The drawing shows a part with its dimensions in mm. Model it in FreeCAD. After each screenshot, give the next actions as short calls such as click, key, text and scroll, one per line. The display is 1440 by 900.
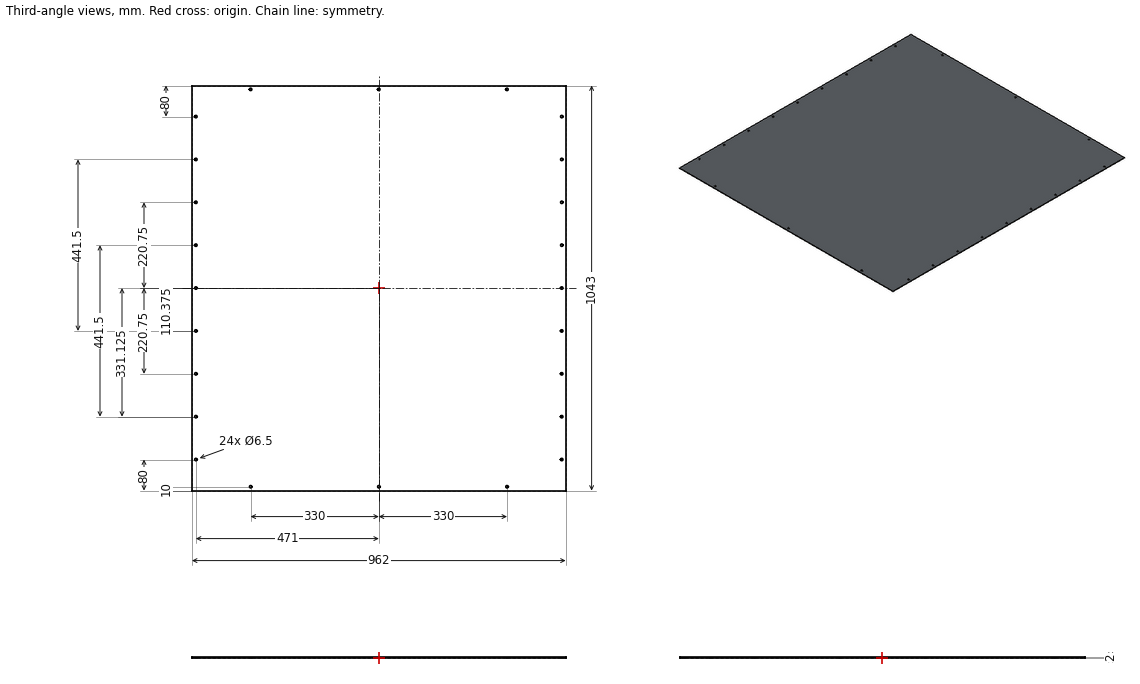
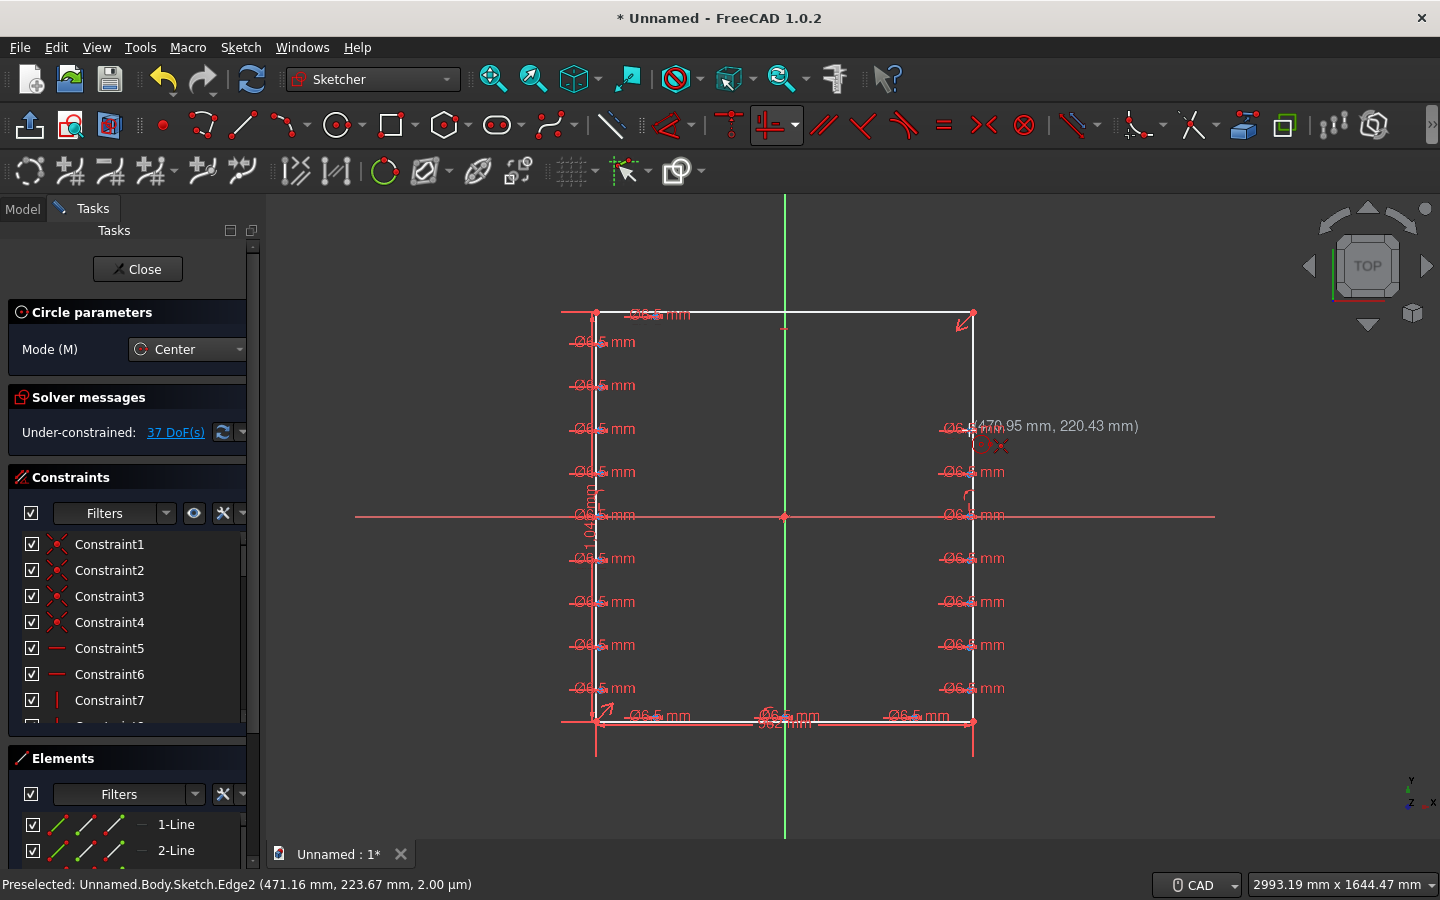
scroll(785, 316, up, 15)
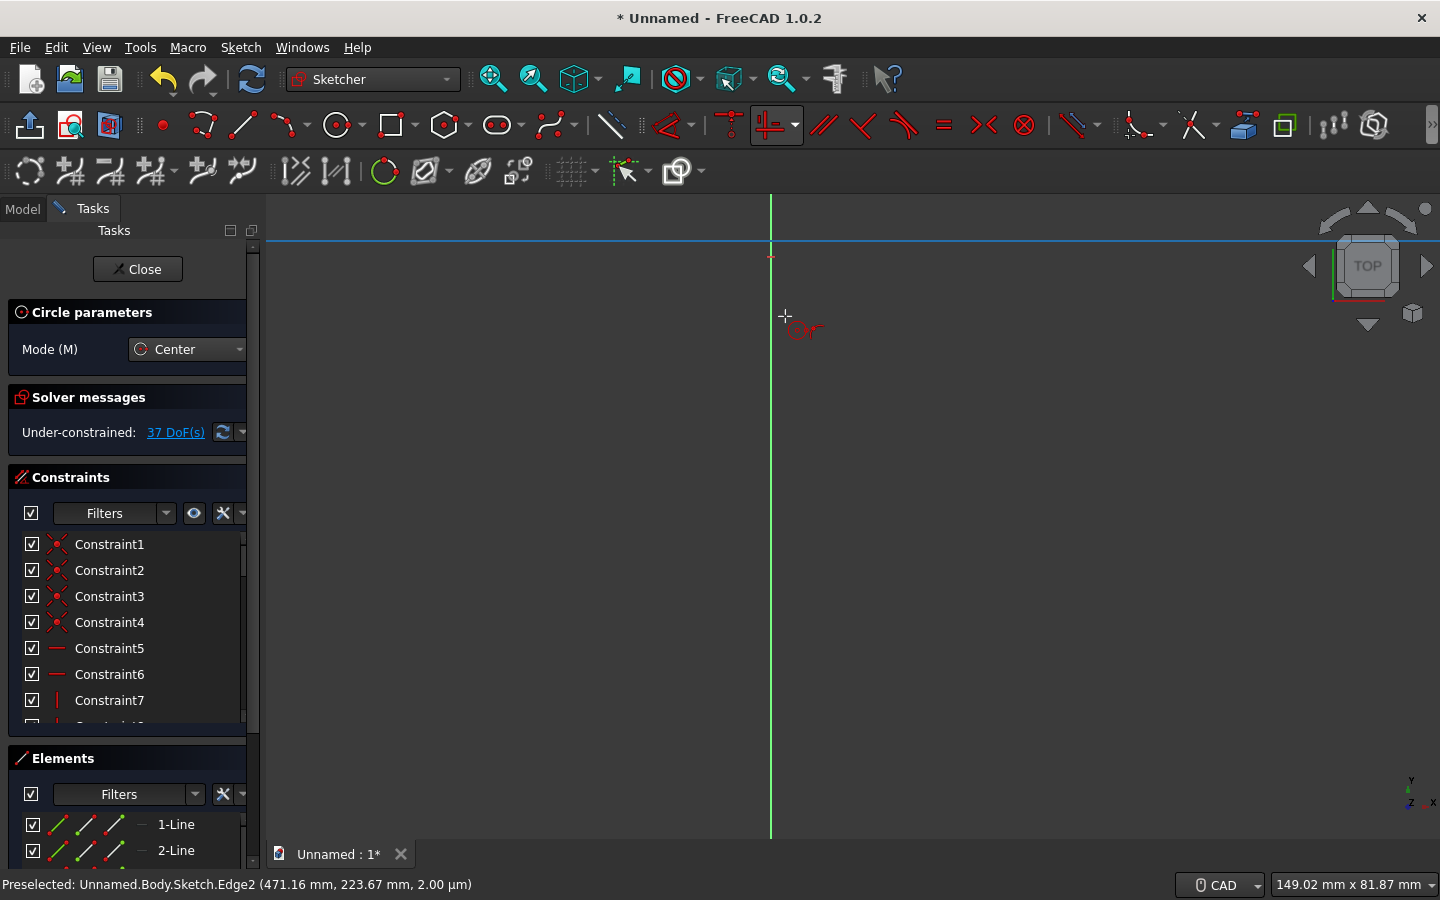
scroll(785, 316, down, 15)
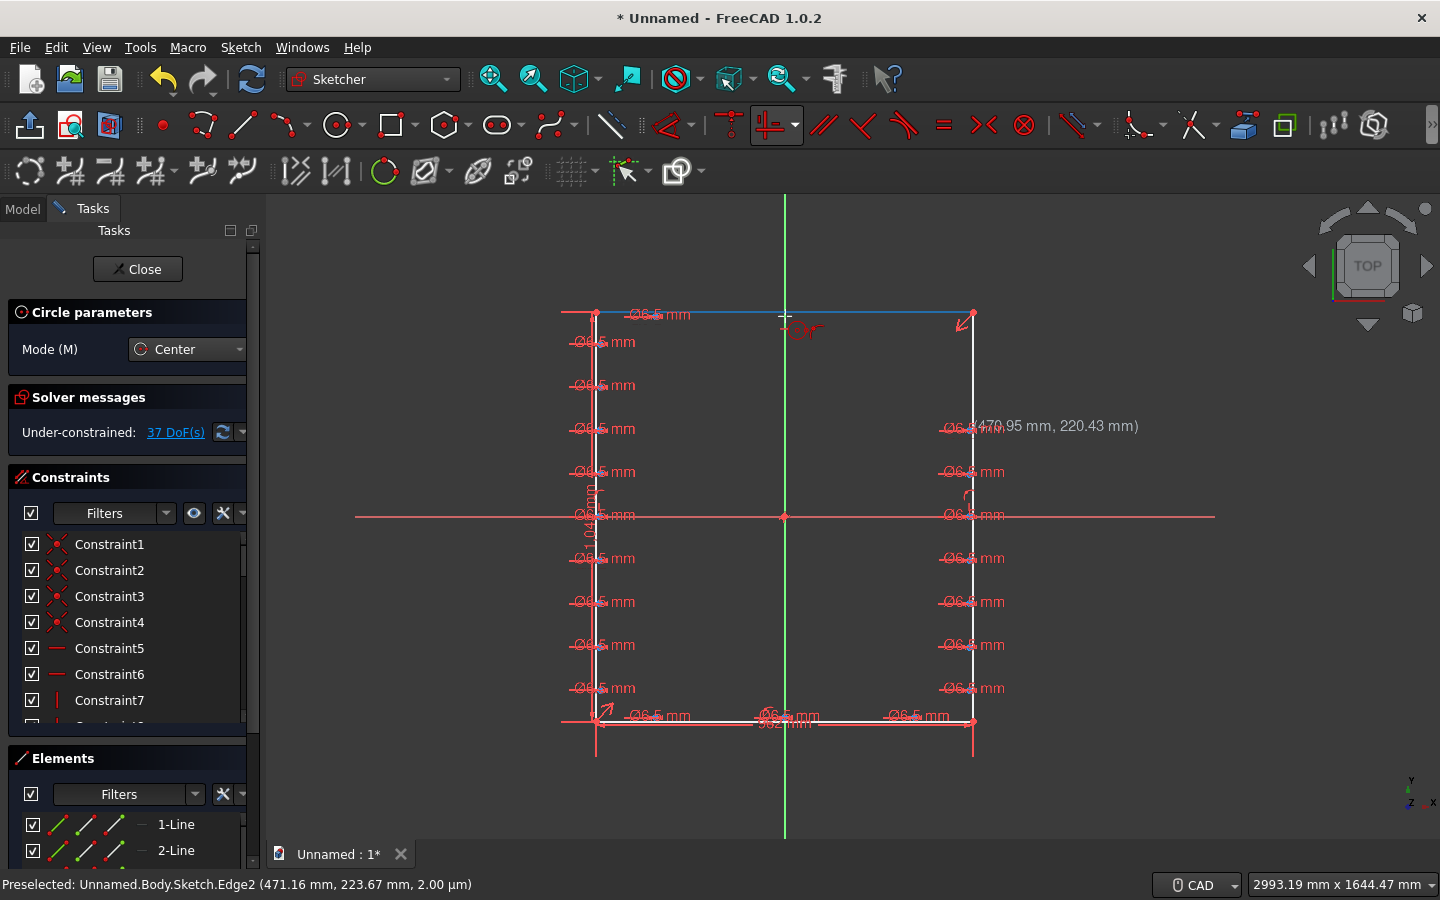
scroll(785, 316, up, 7)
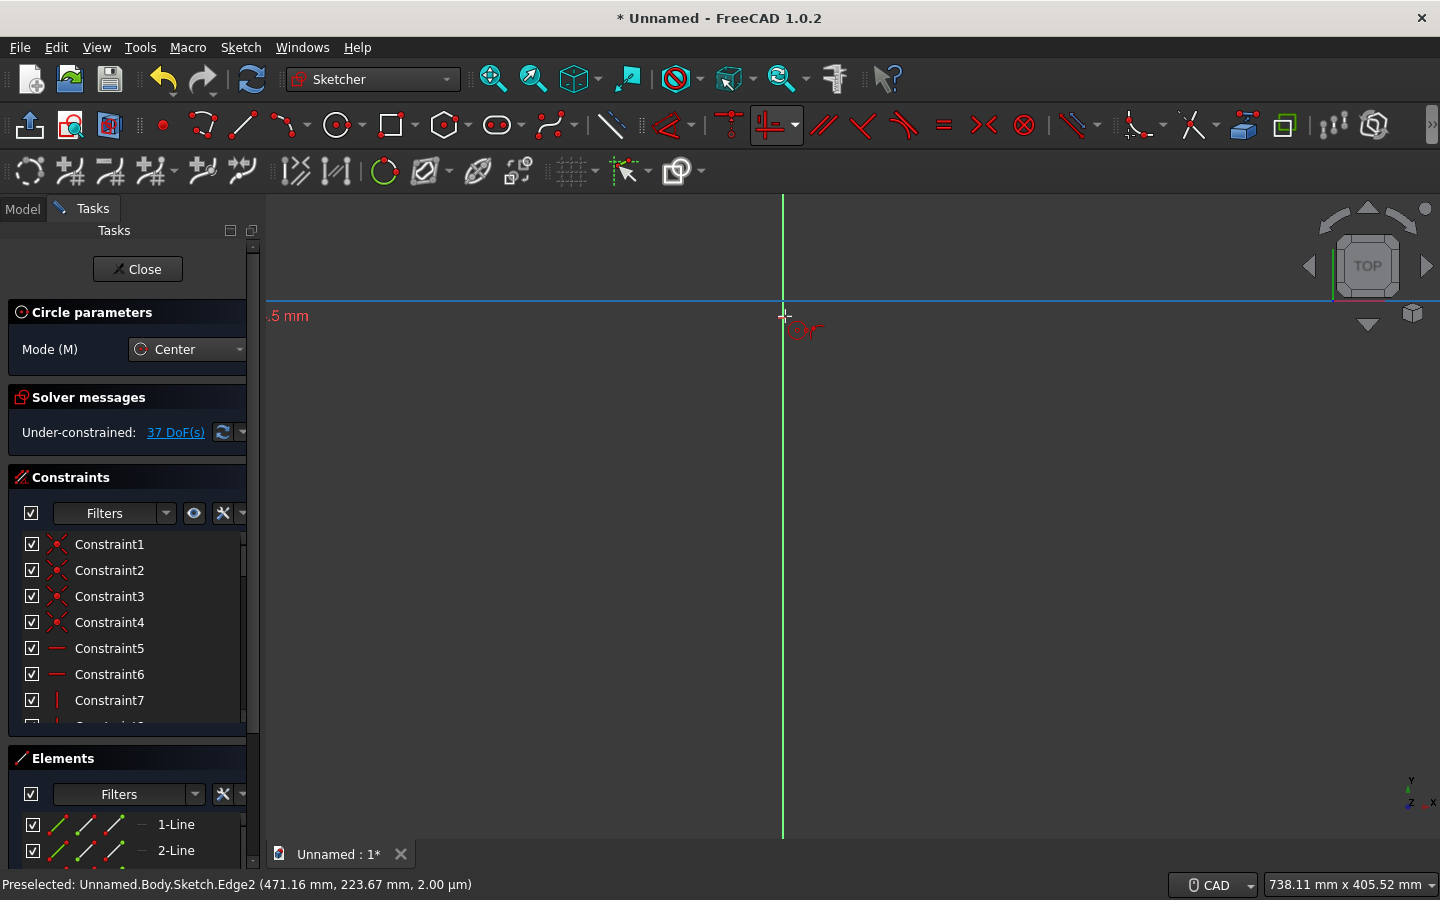
click(783, 317)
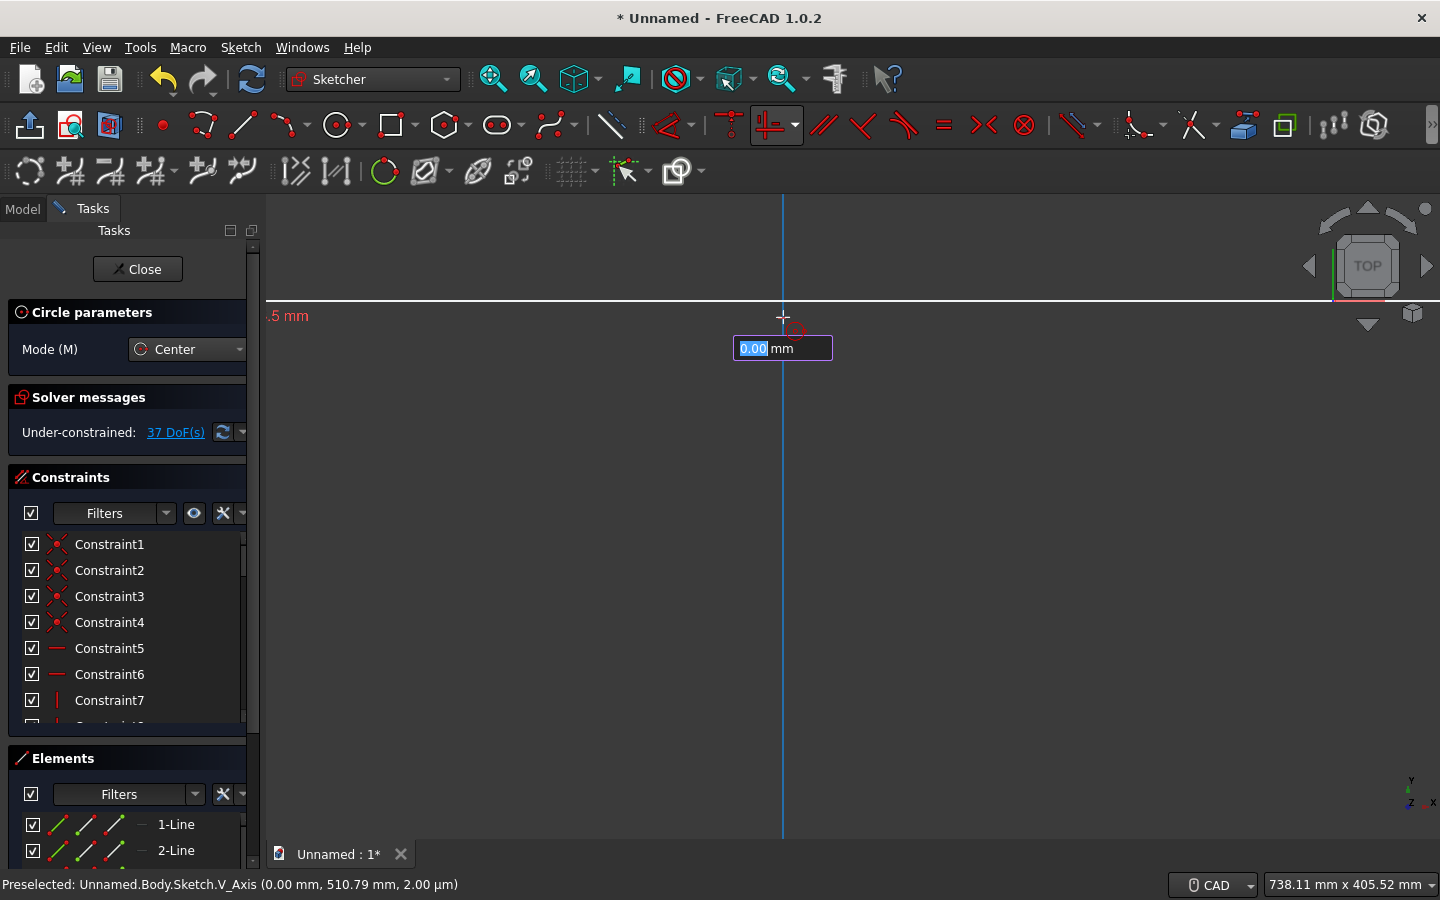
scroll(787, 315, up, 6)
move(787, 315)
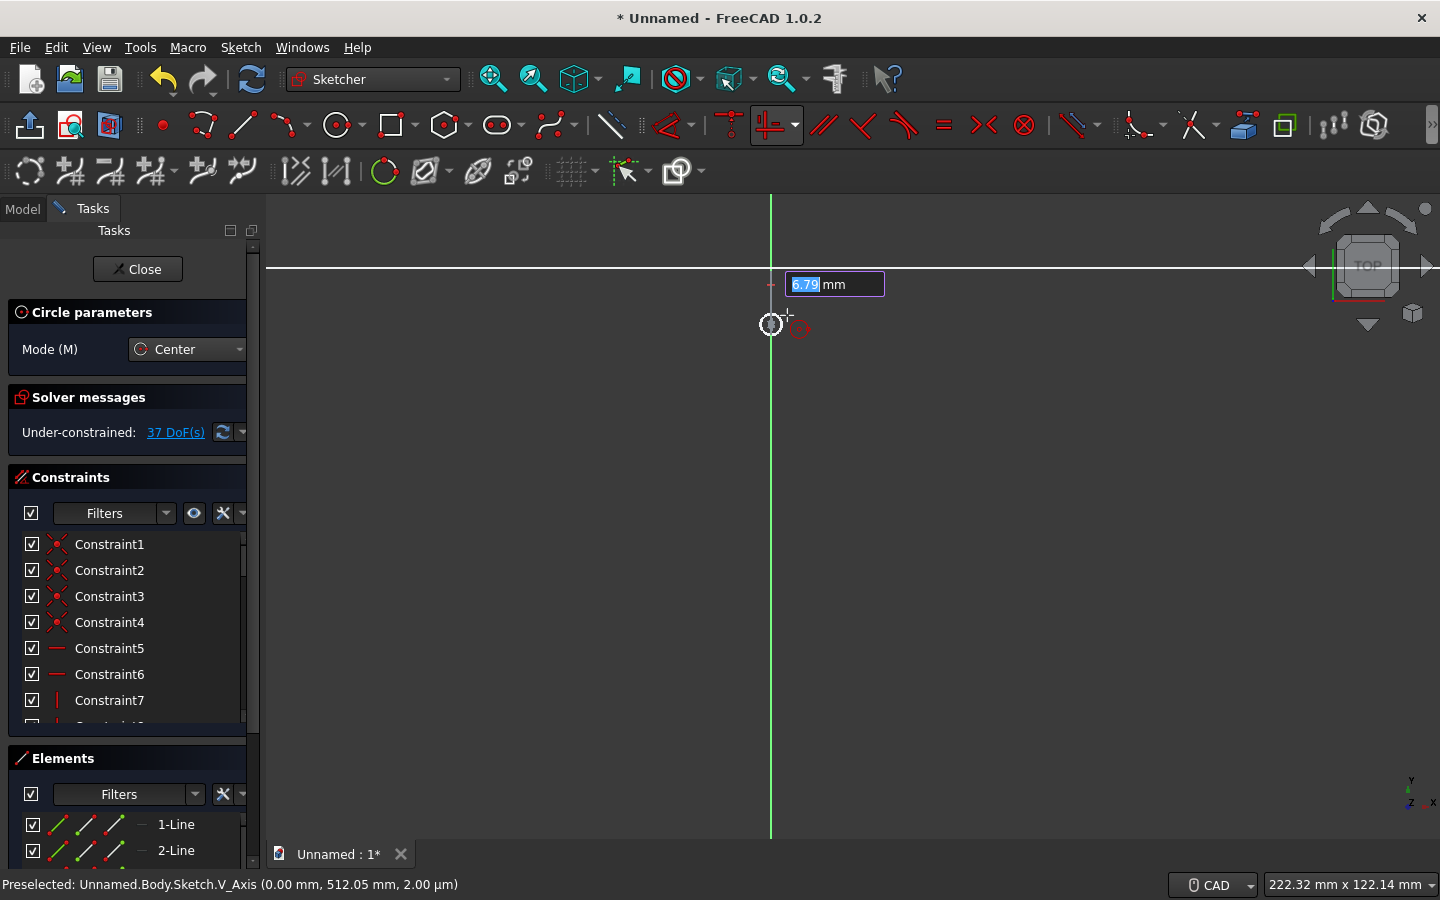
text(6.5)
key(Return)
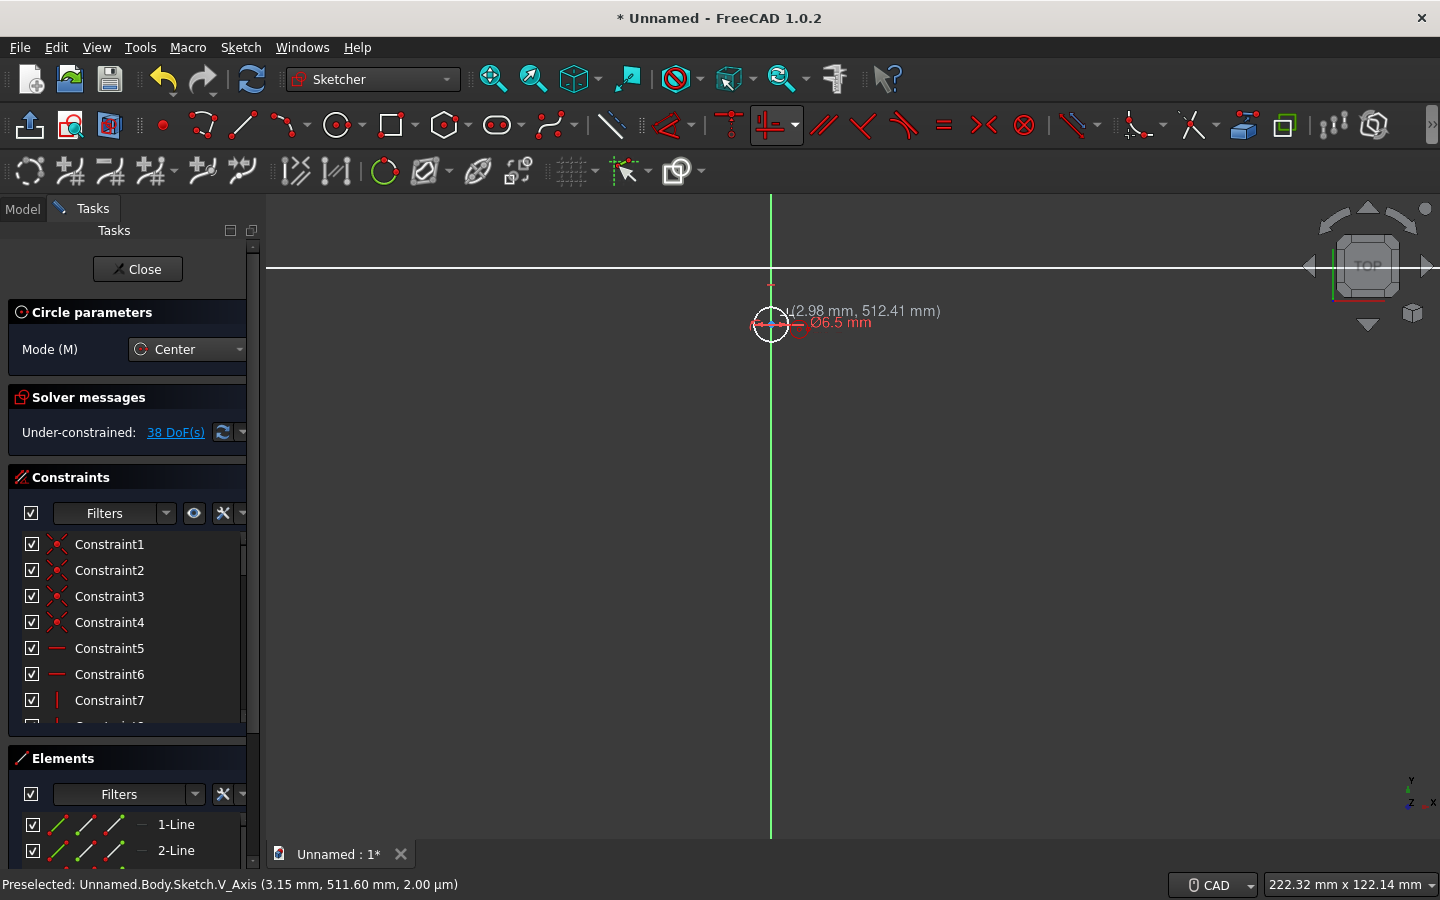
scroll(786, 315, down, 13)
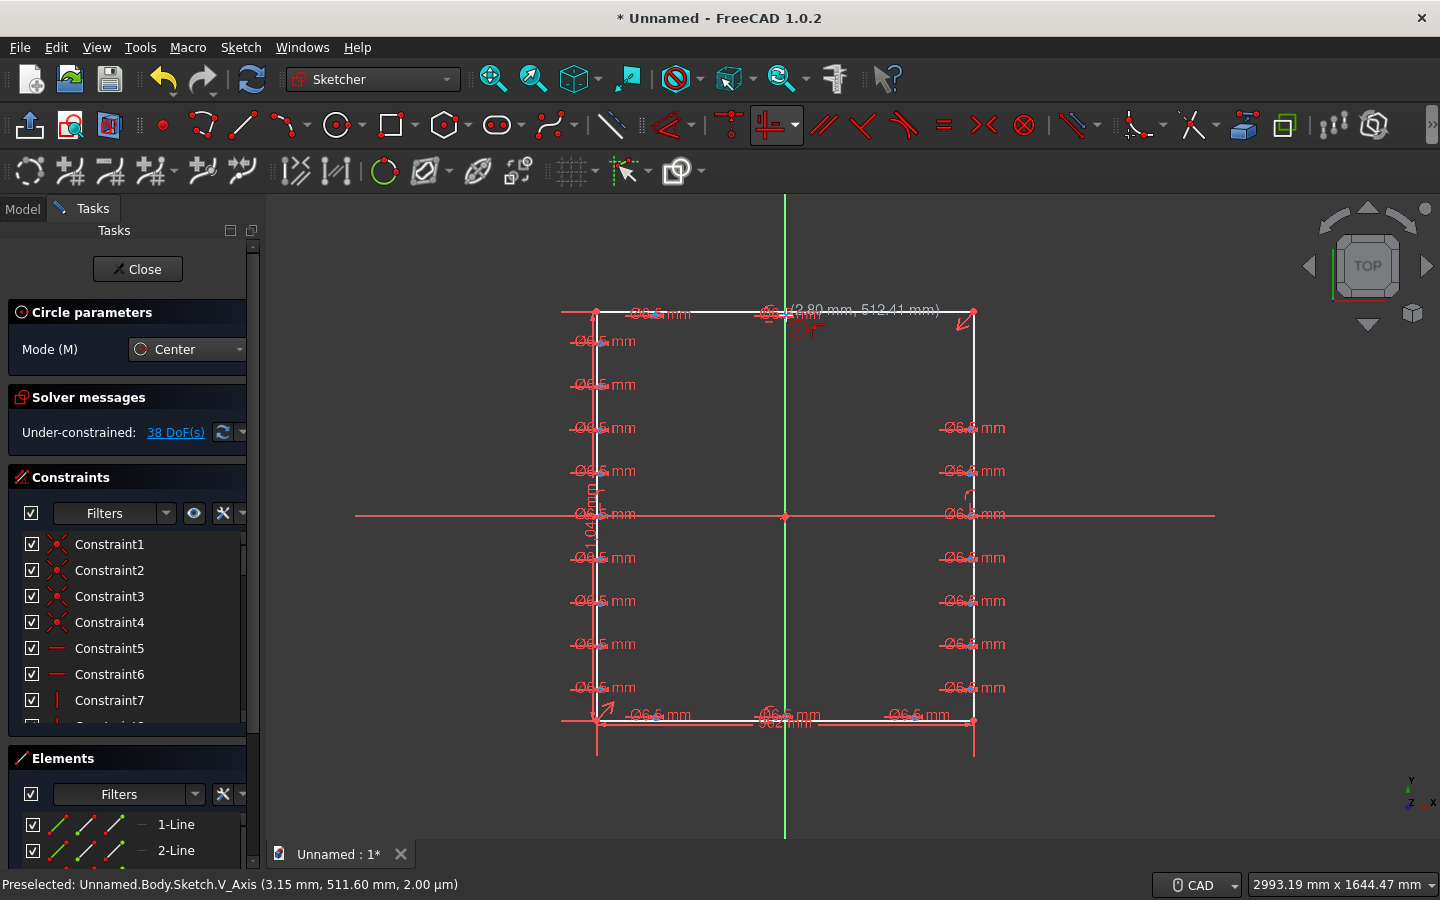
scroll(970, 386, up, 15)